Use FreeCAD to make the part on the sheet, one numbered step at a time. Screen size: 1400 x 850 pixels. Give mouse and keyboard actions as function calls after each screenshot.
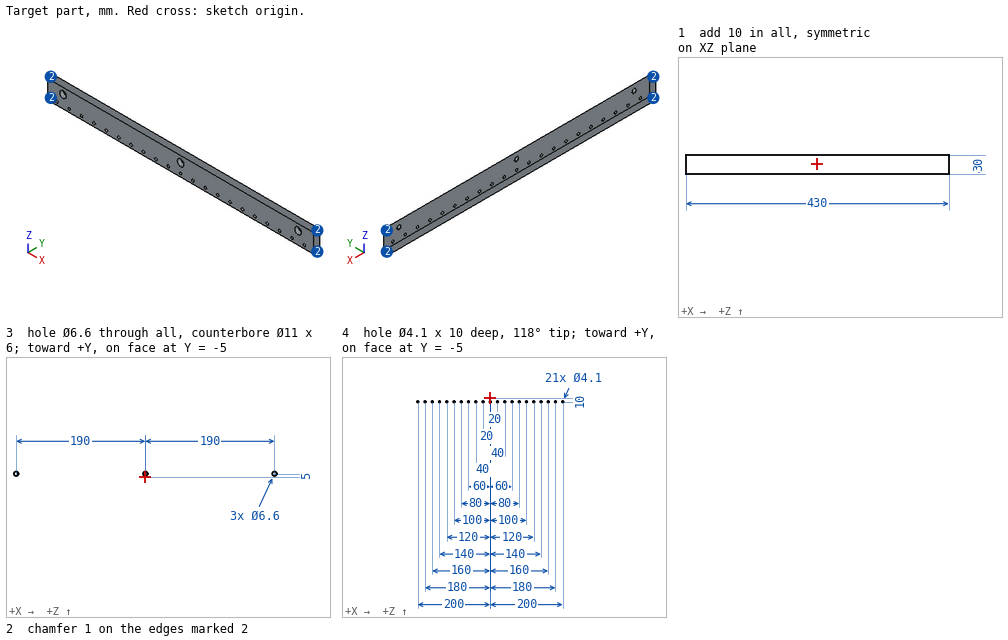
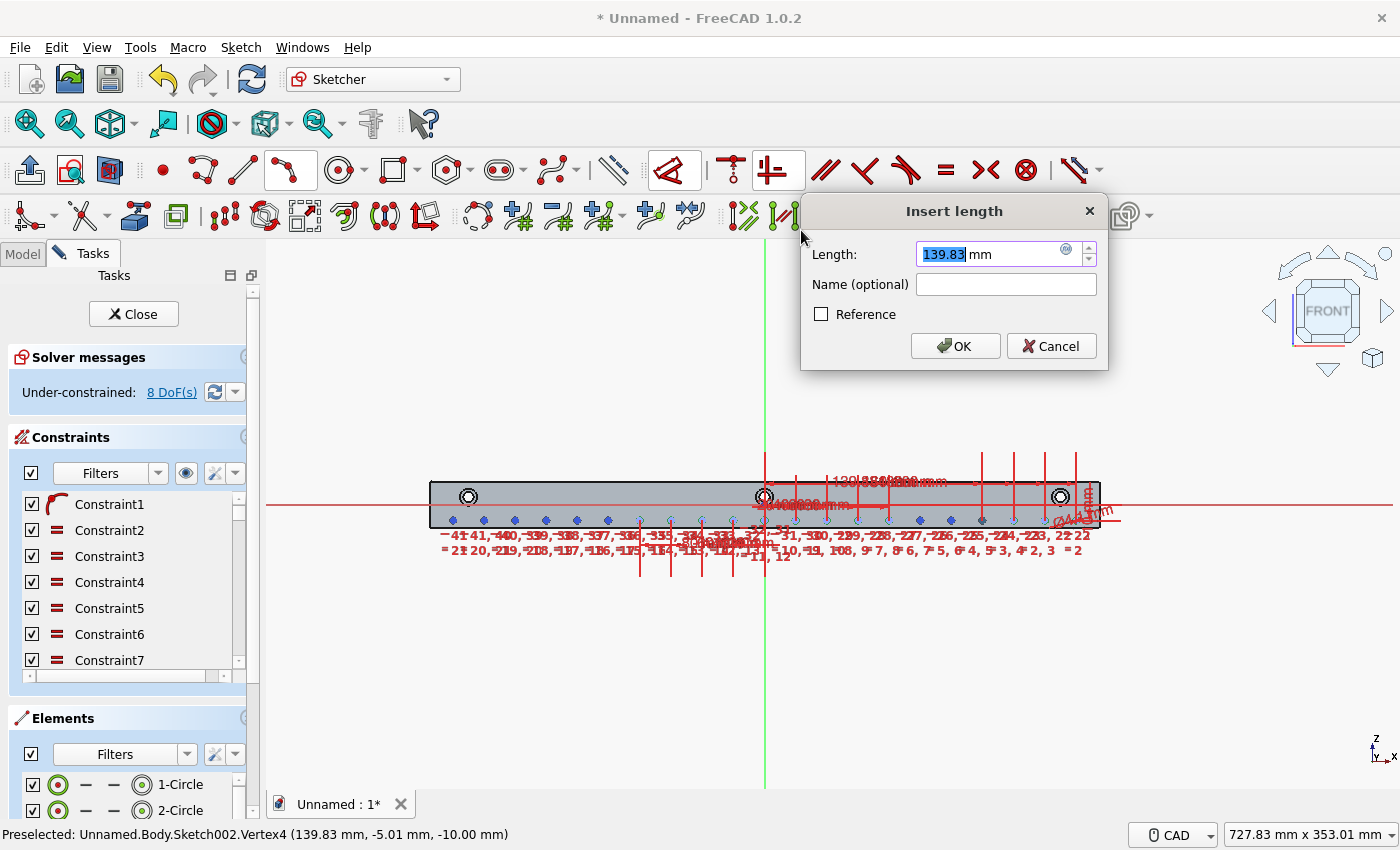
text(140)
key(Return)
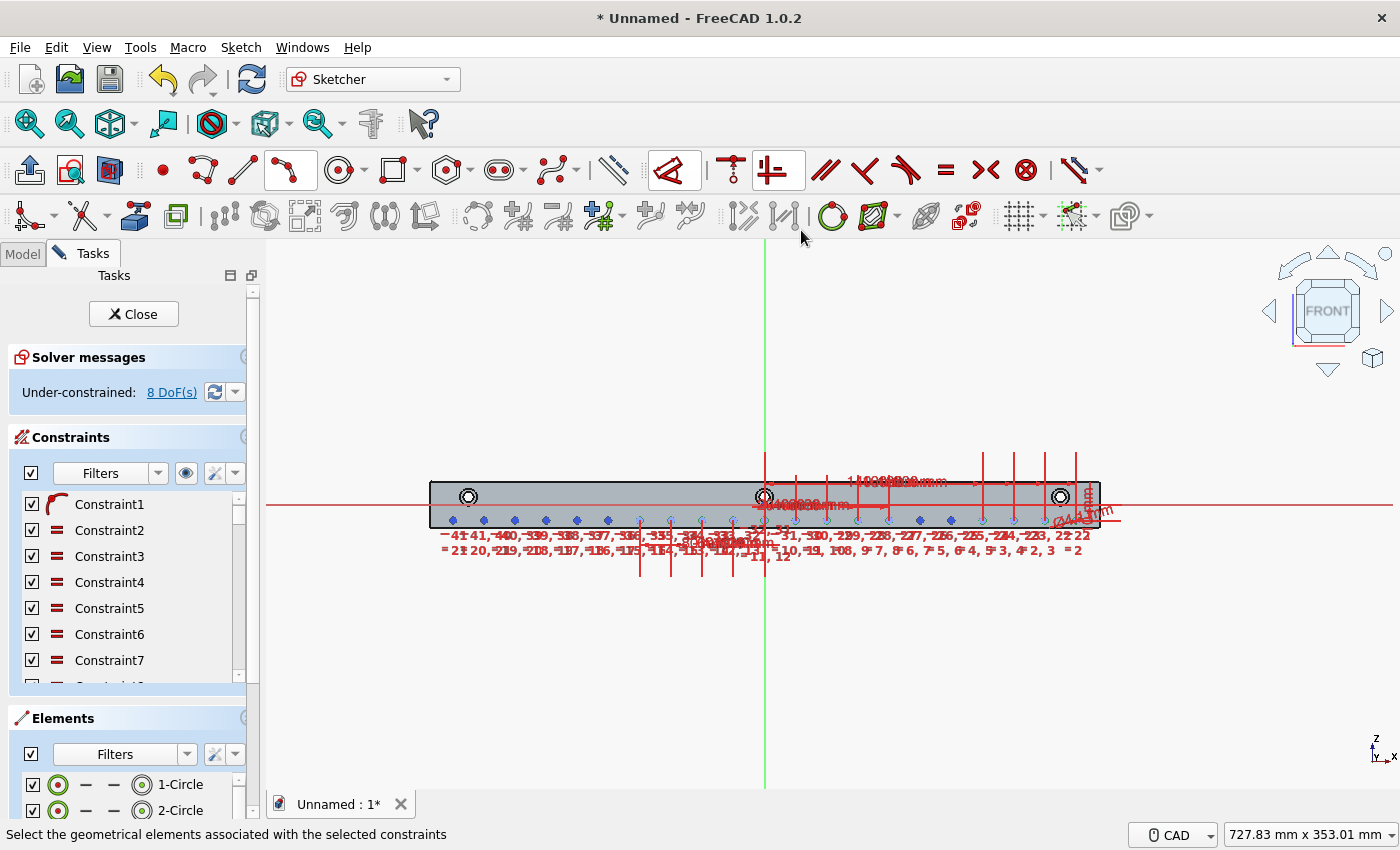
click(951, 521)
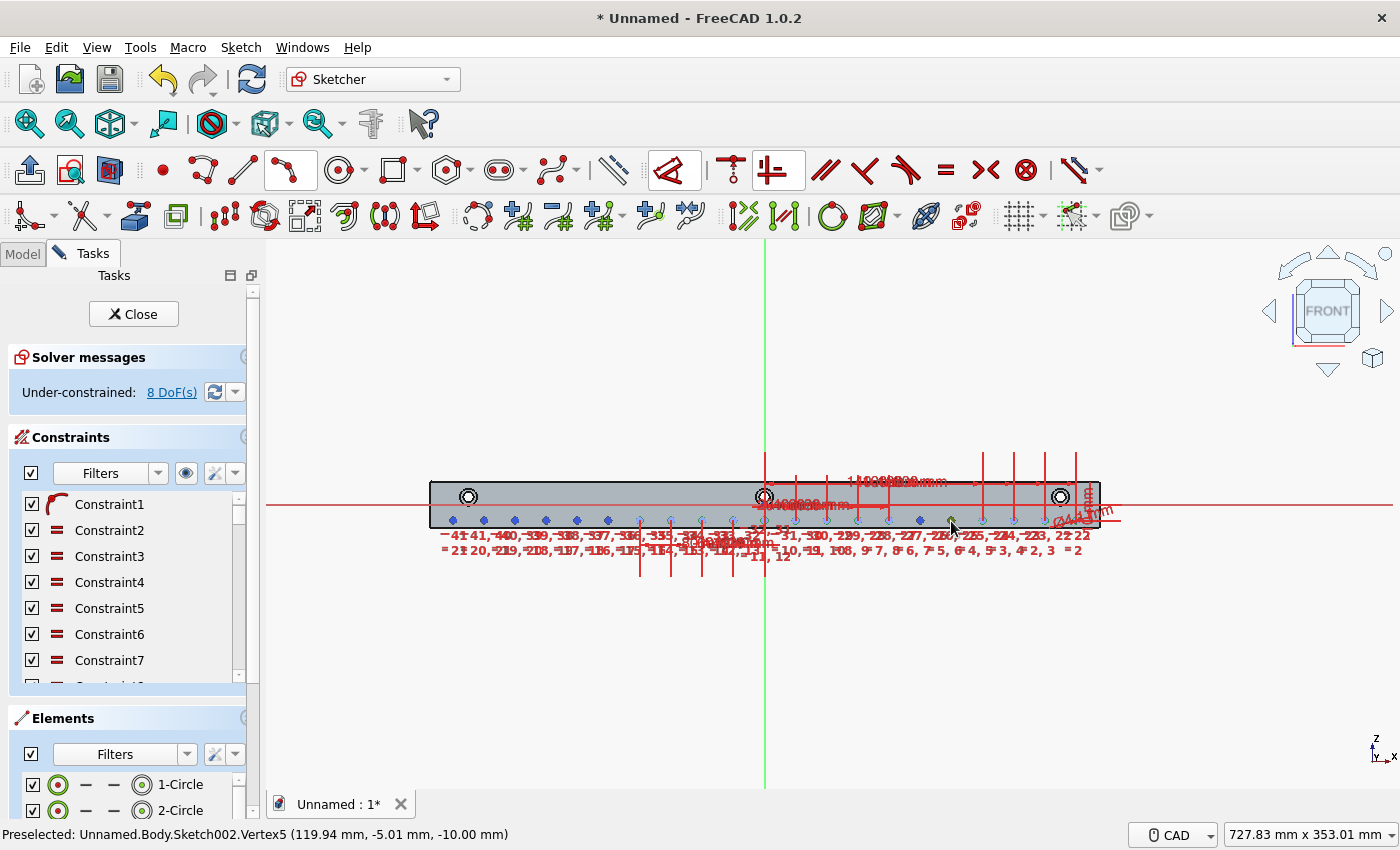
key(l)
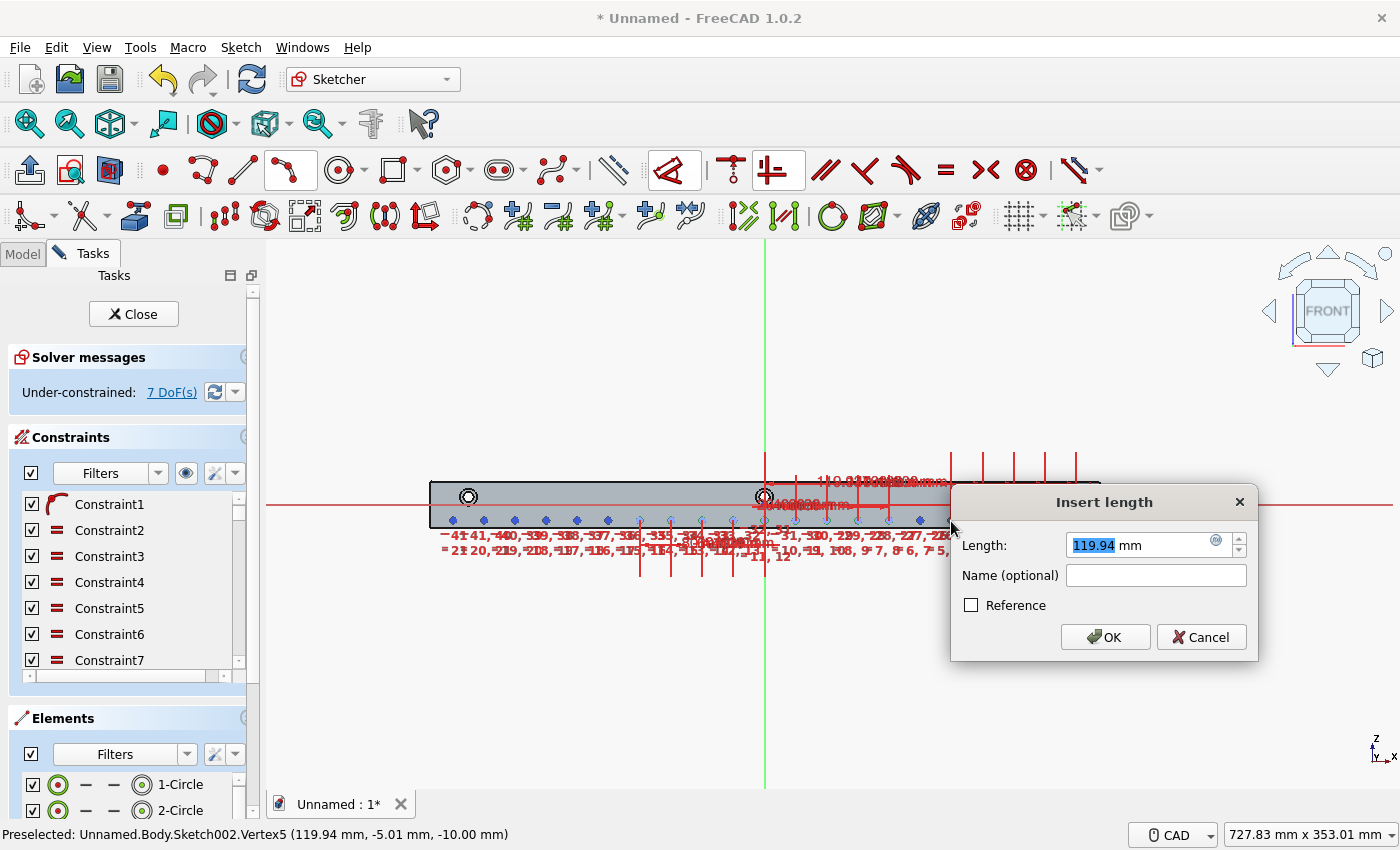
text(120)
key(Return)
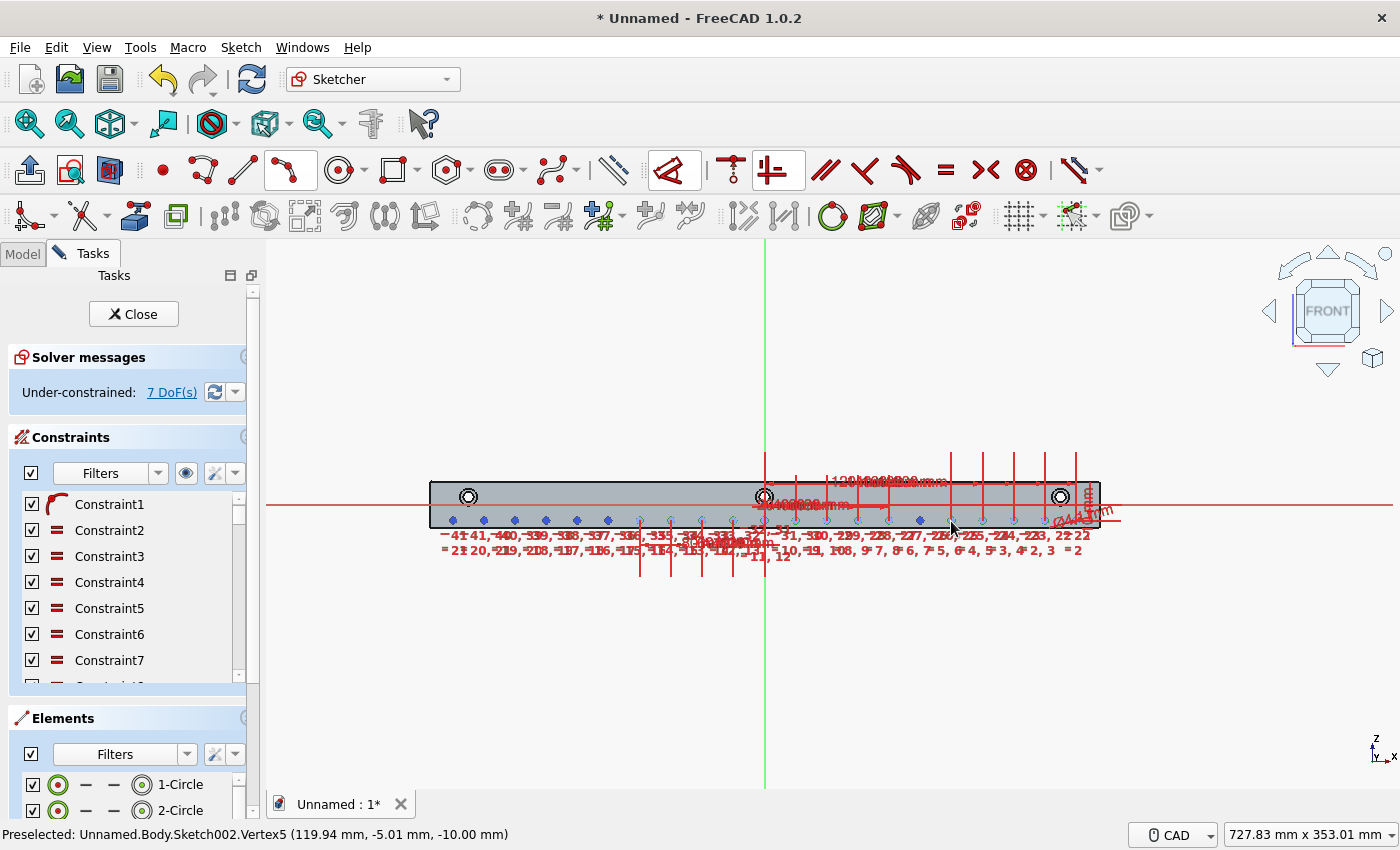
click(920, 521)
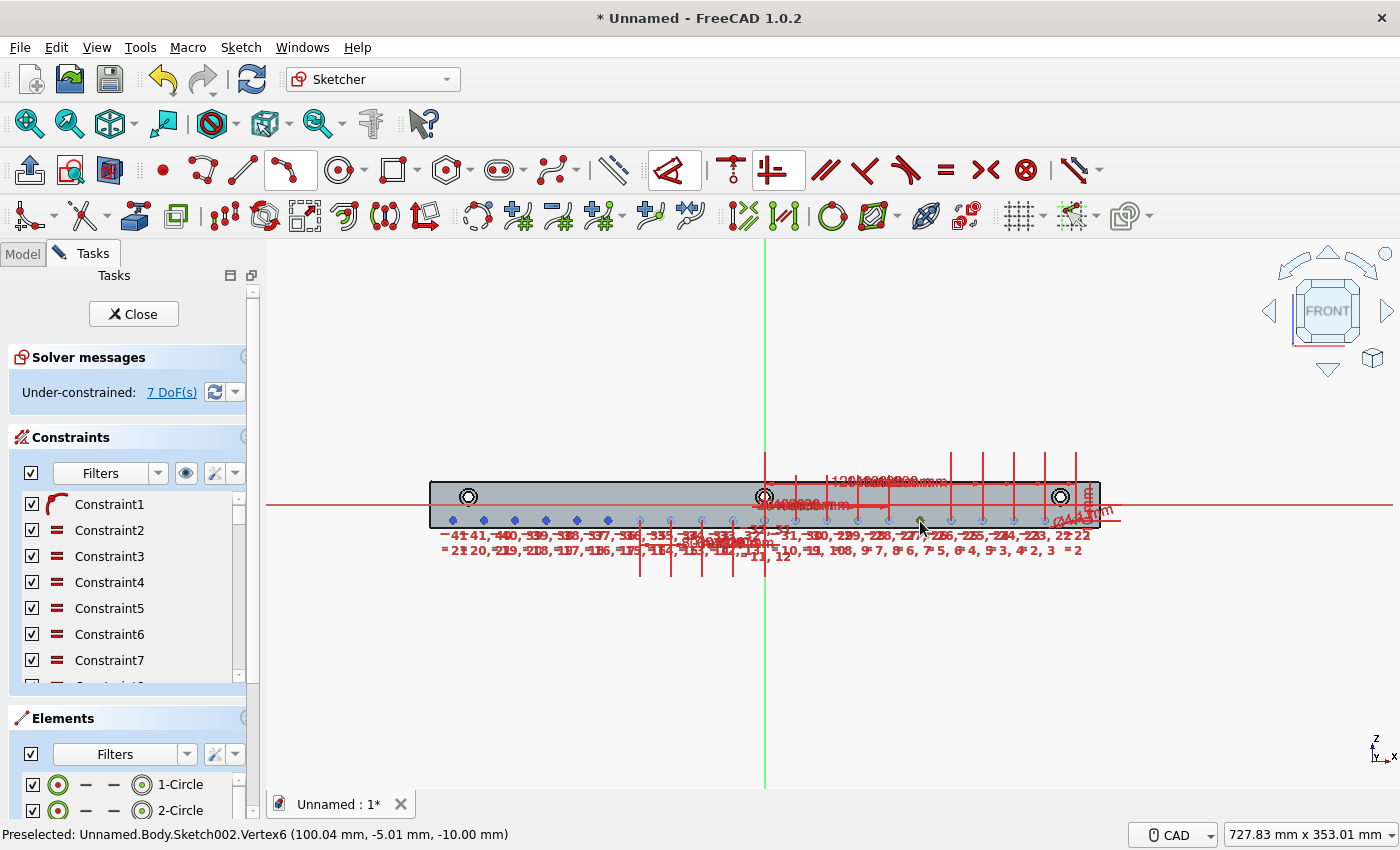
click(696, 170)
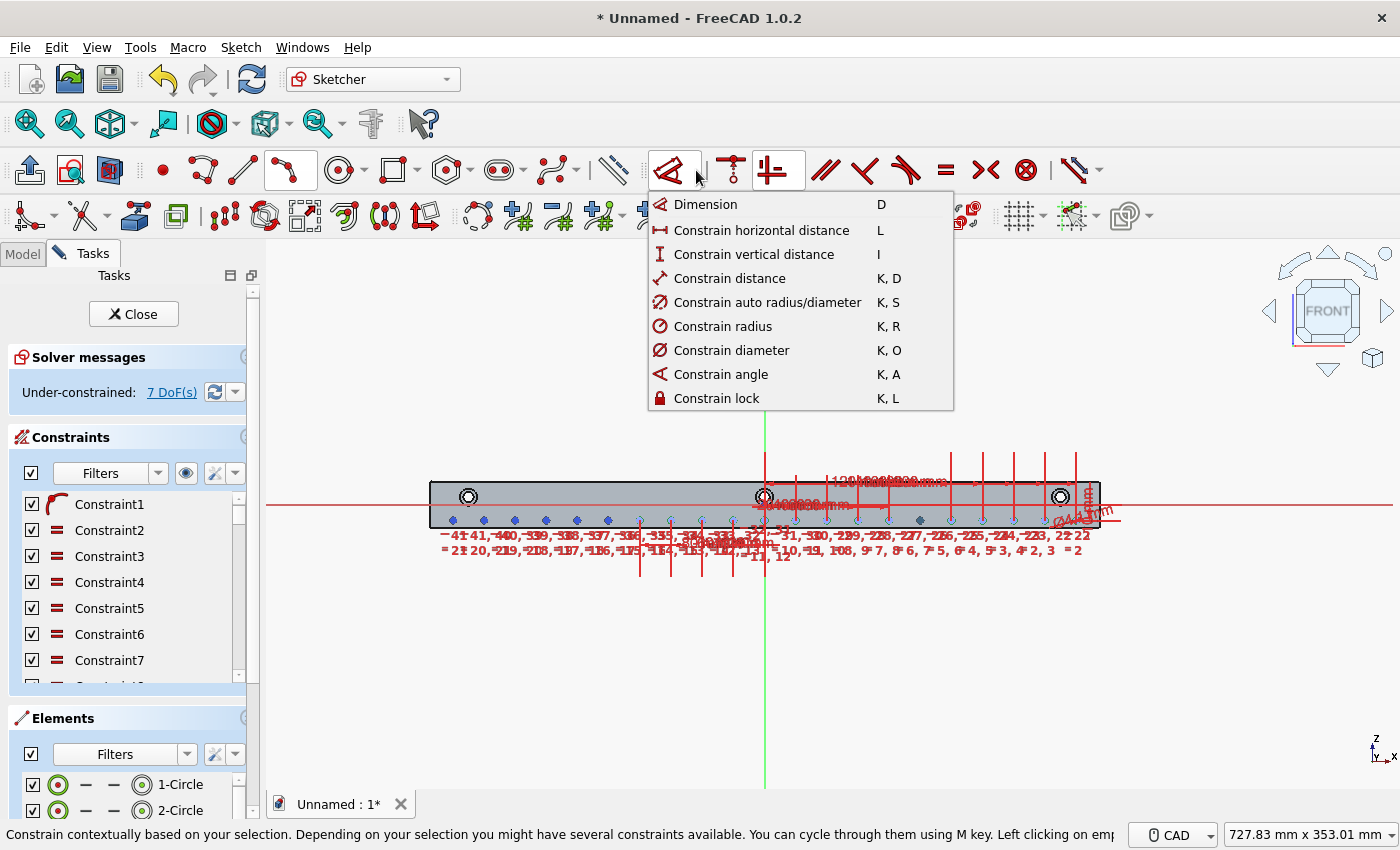
click(801, 230)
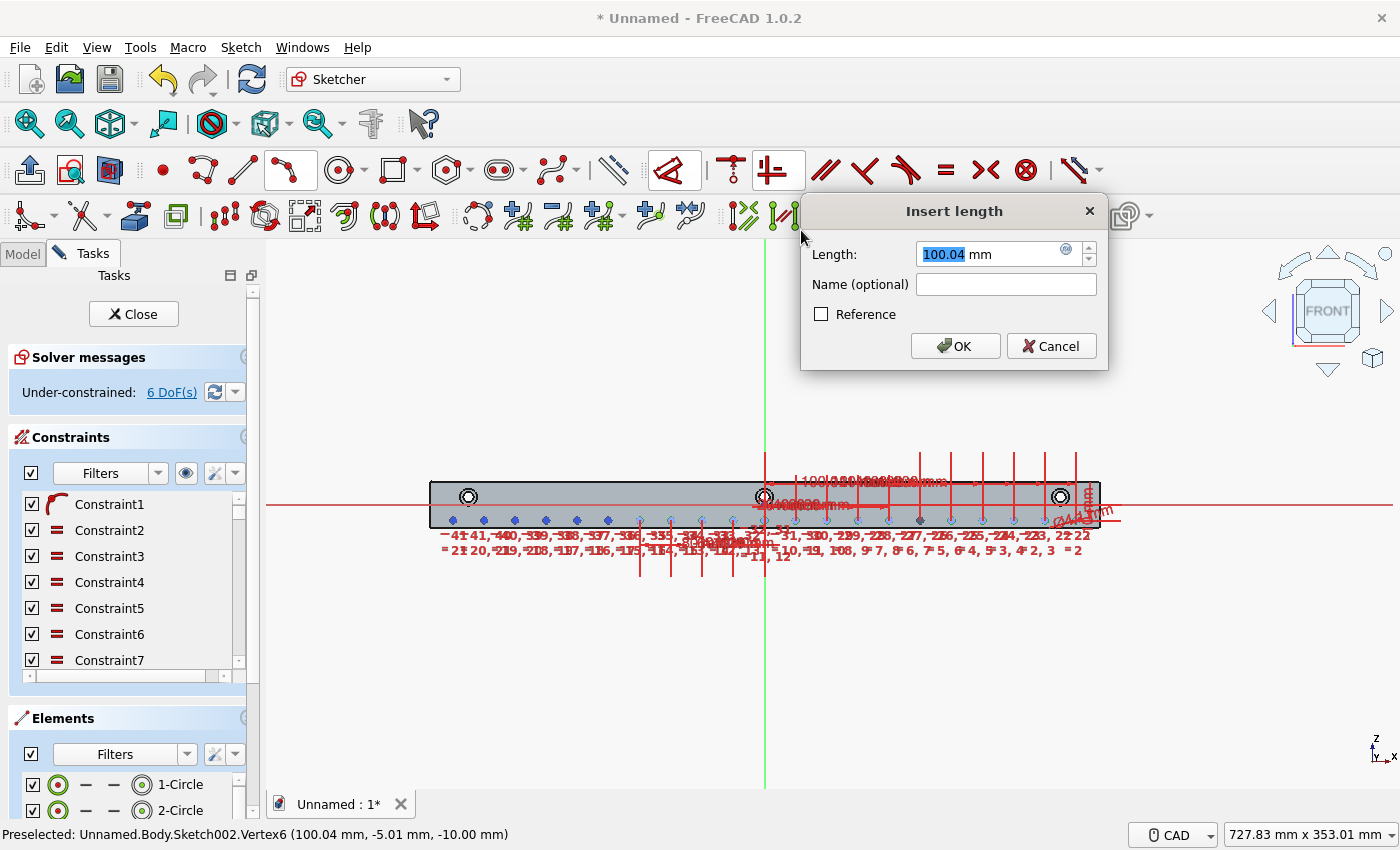
text(100)
key(Return)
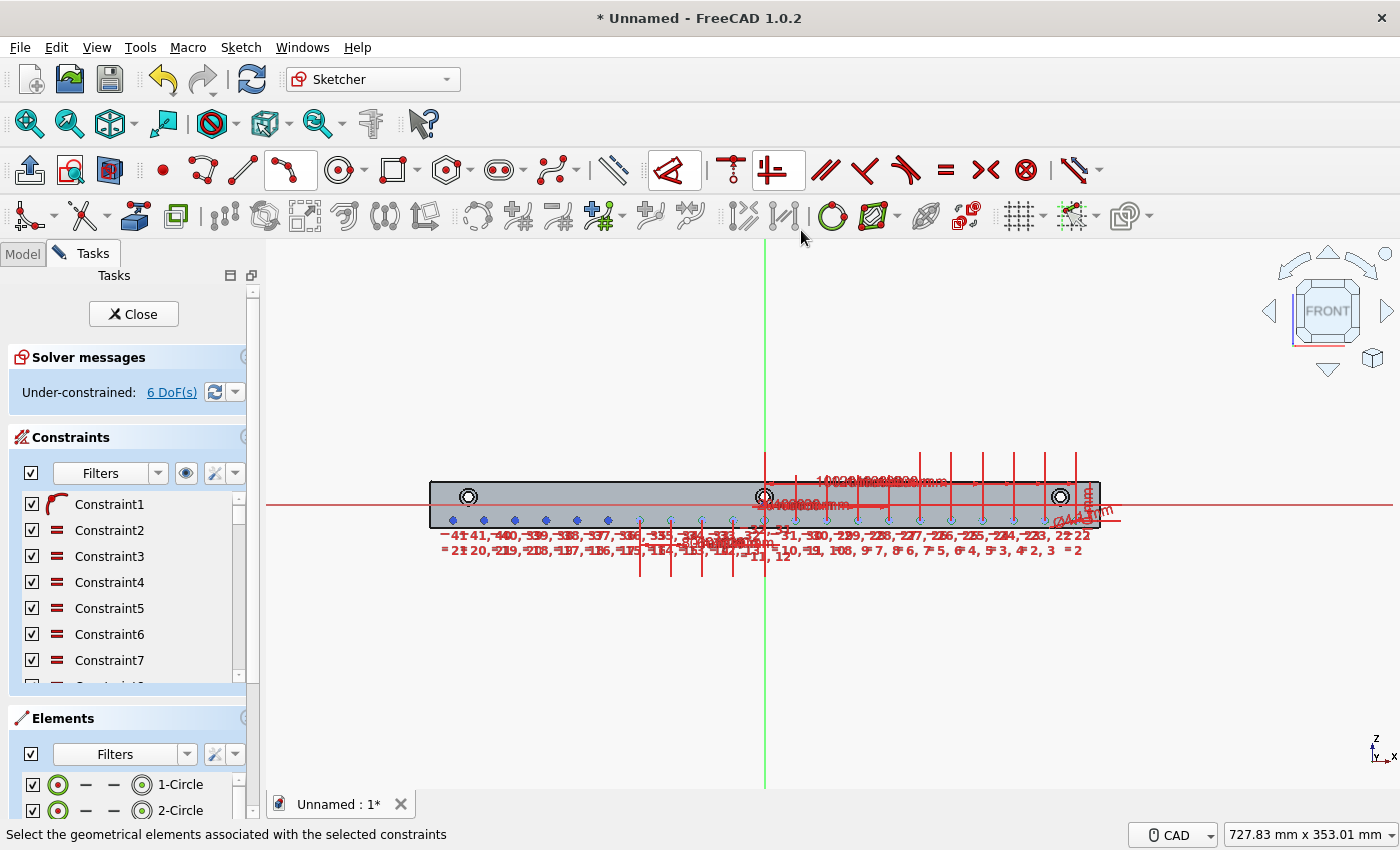
click(608, 521)